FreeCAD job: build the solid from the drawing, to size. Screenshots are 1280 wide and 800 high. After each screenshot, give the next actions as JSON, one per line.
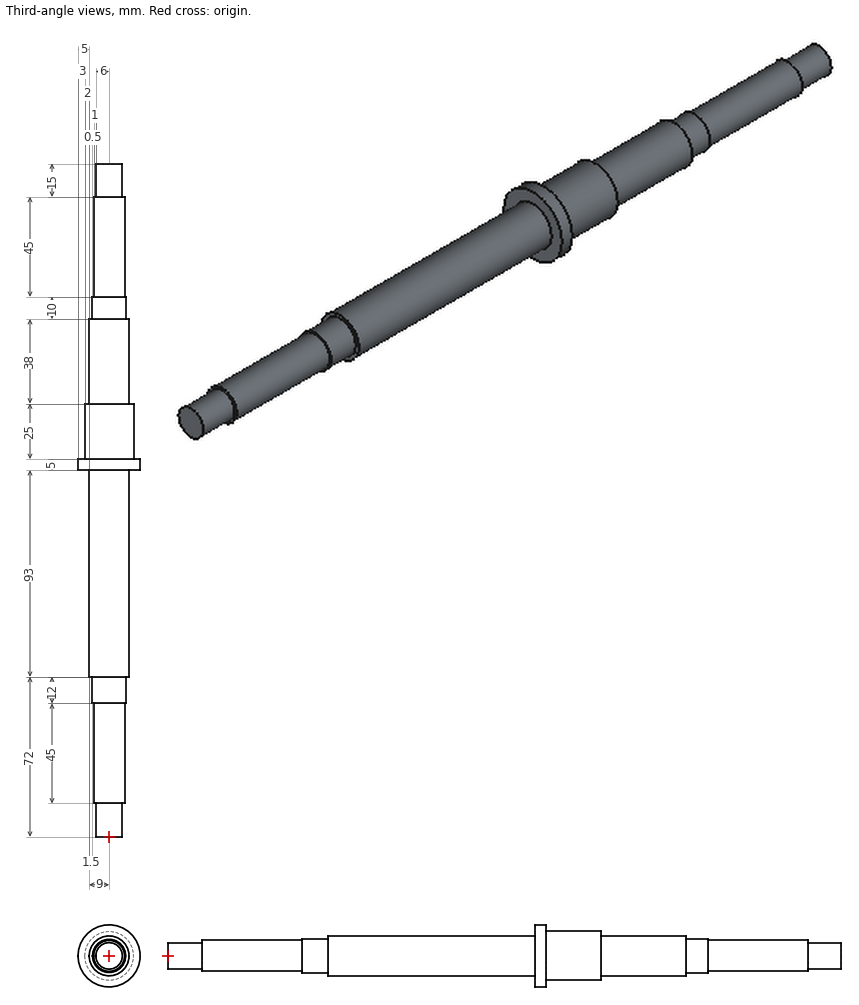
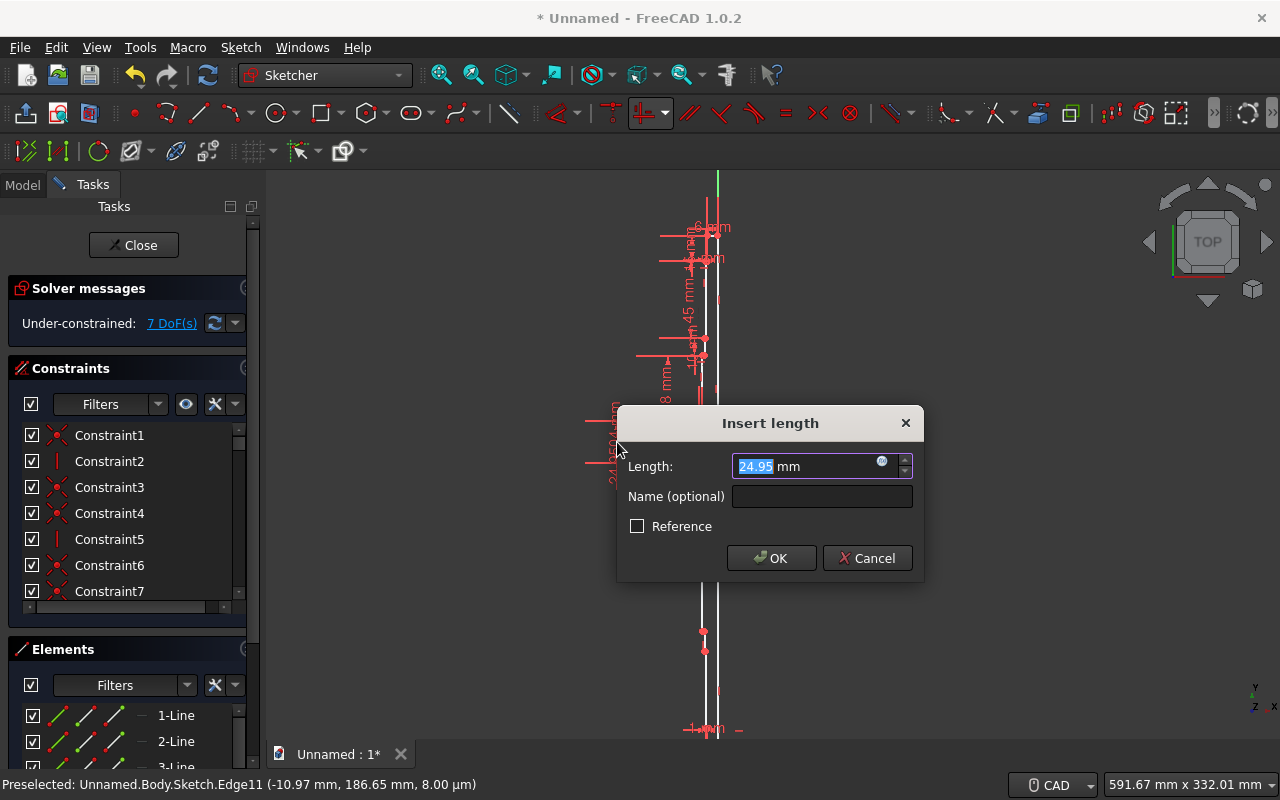
{"action": "type", "text": "25"}
{"action": "key", "text": "Return"}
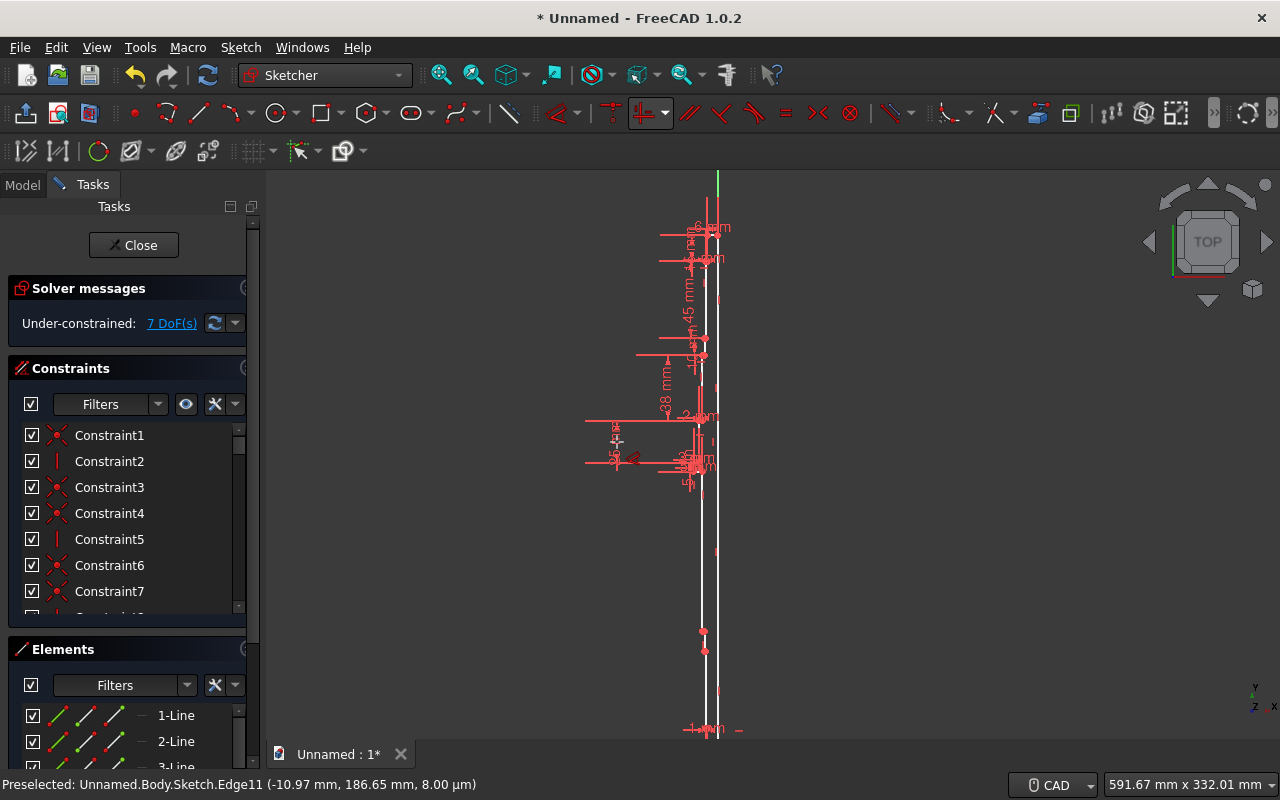
{"action": "left_click", "coordinate": [702, 520]}
{"action": "left_click", "coordinate": [668, 552]}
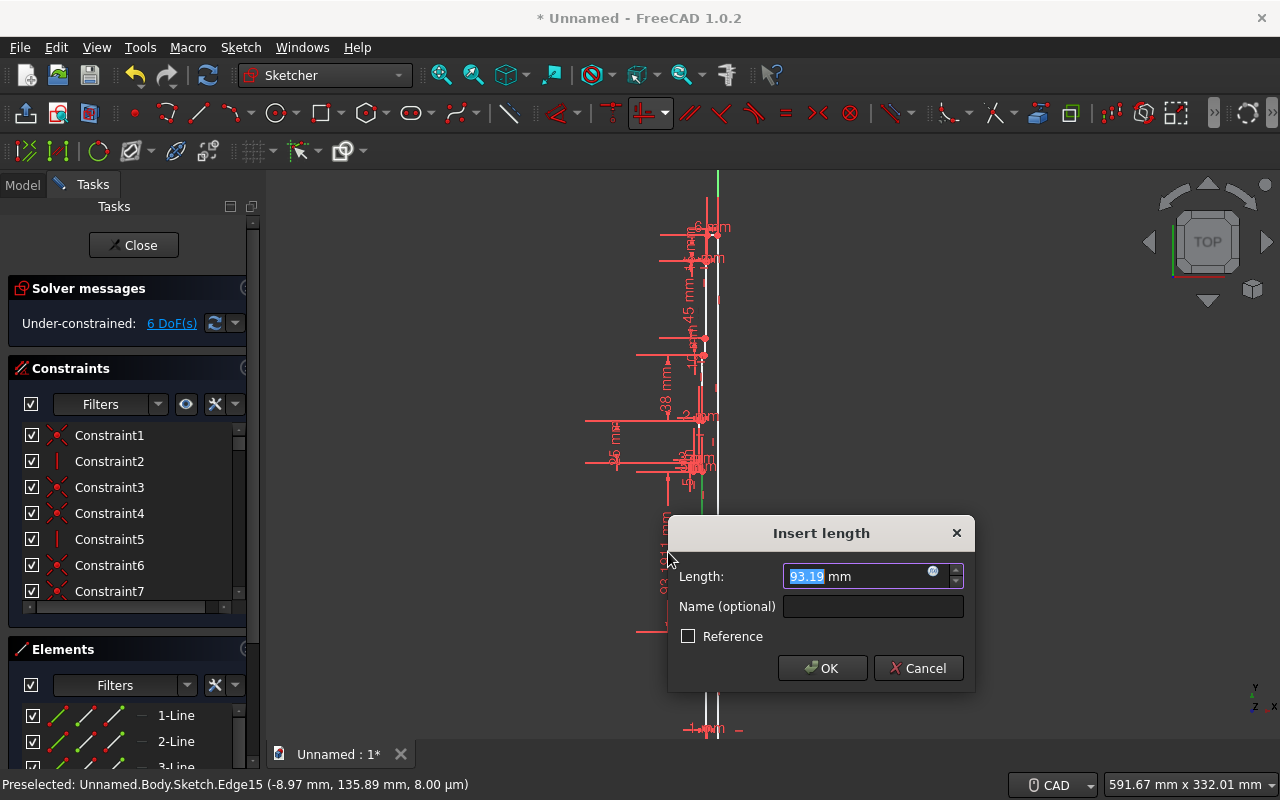
{"action": "type", "text": "93"}
{"action": "key", "text": "Return"}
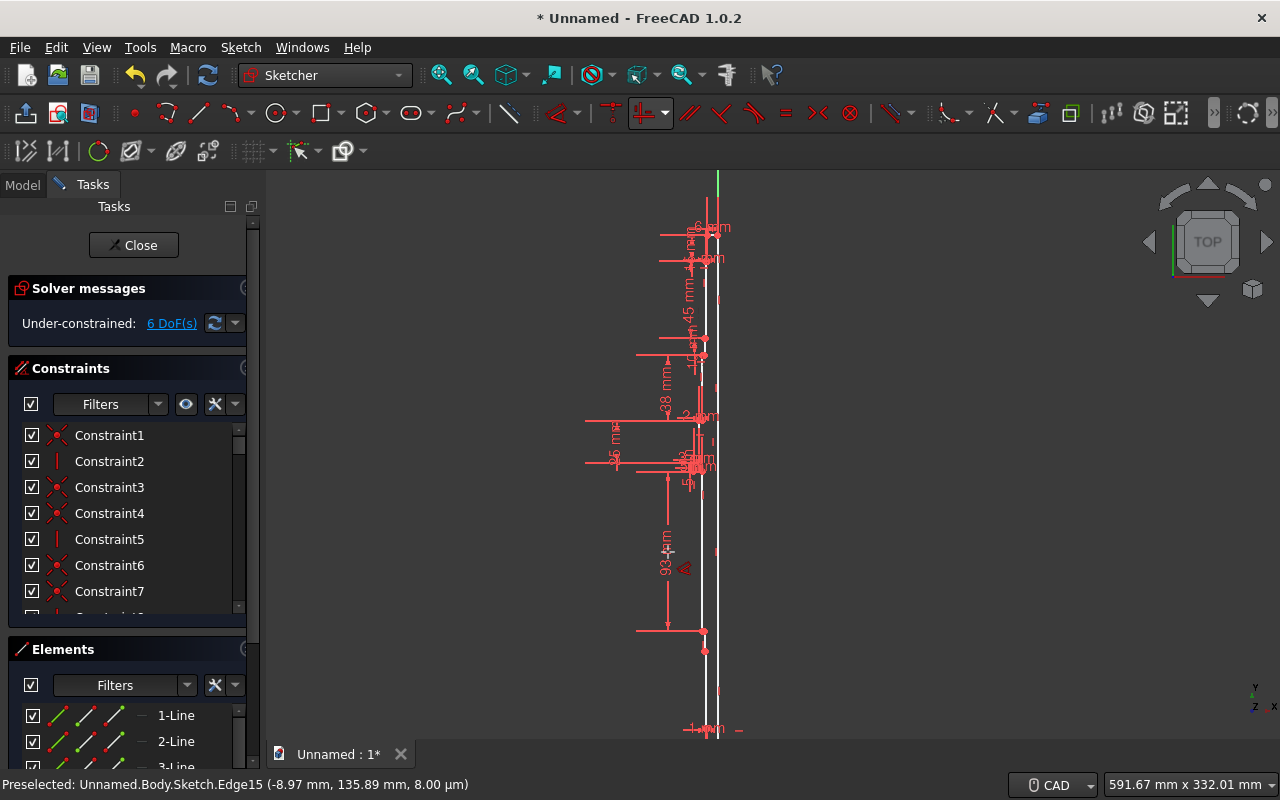
{"action": "scroll", "coordinate": [705, 642], "scroll_direction": "up", "scroll_amount": 4}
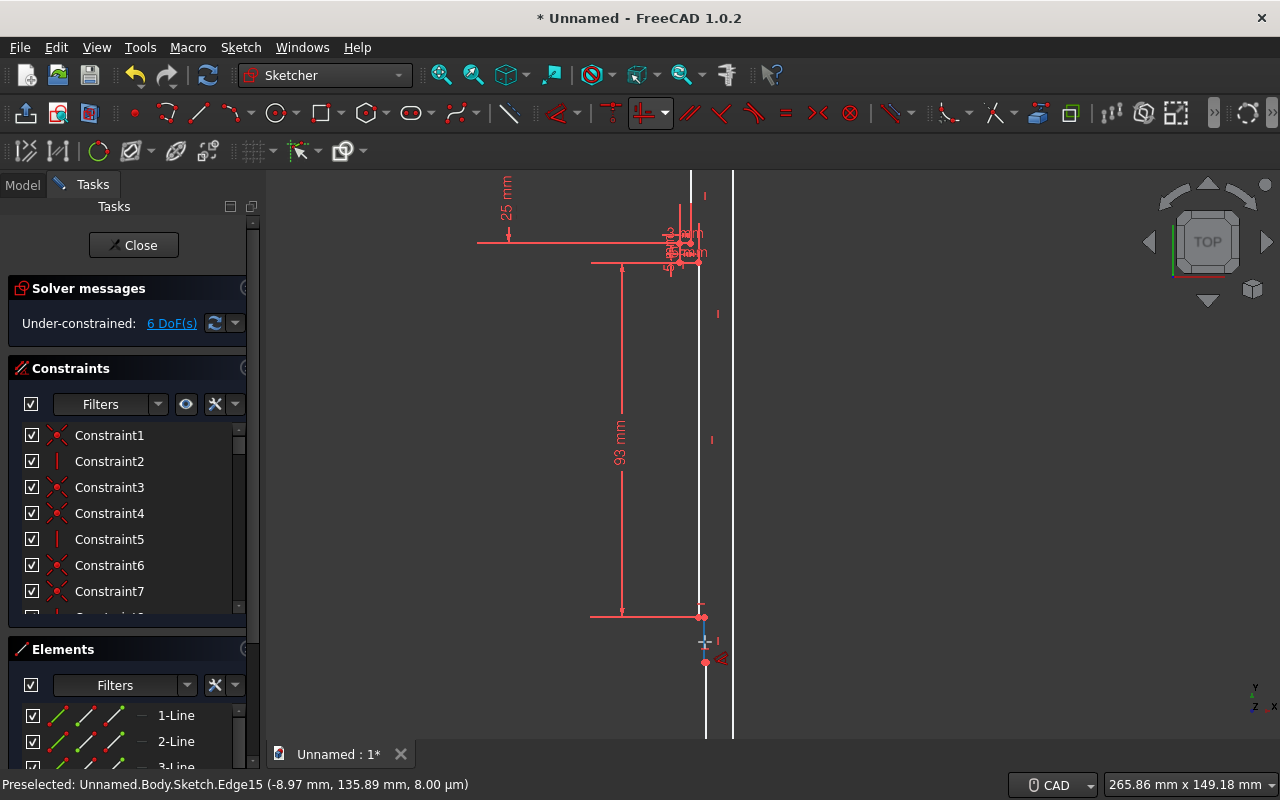
{"action": "left_click", "coordinate": [704, 640]}
{"action": "left_click", "coordinate": [670, 640]}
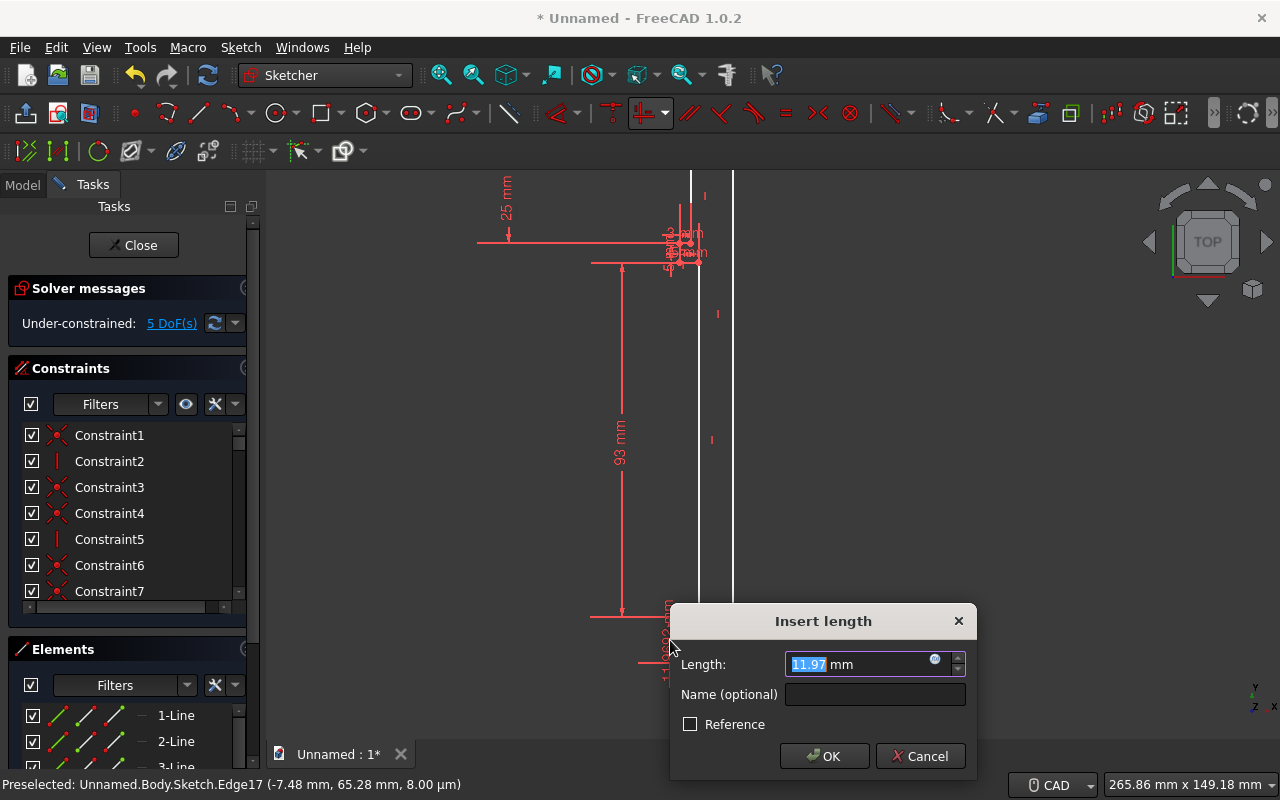
{"action": "type", "text": "12"}
{"action": "key", "text": "Return"}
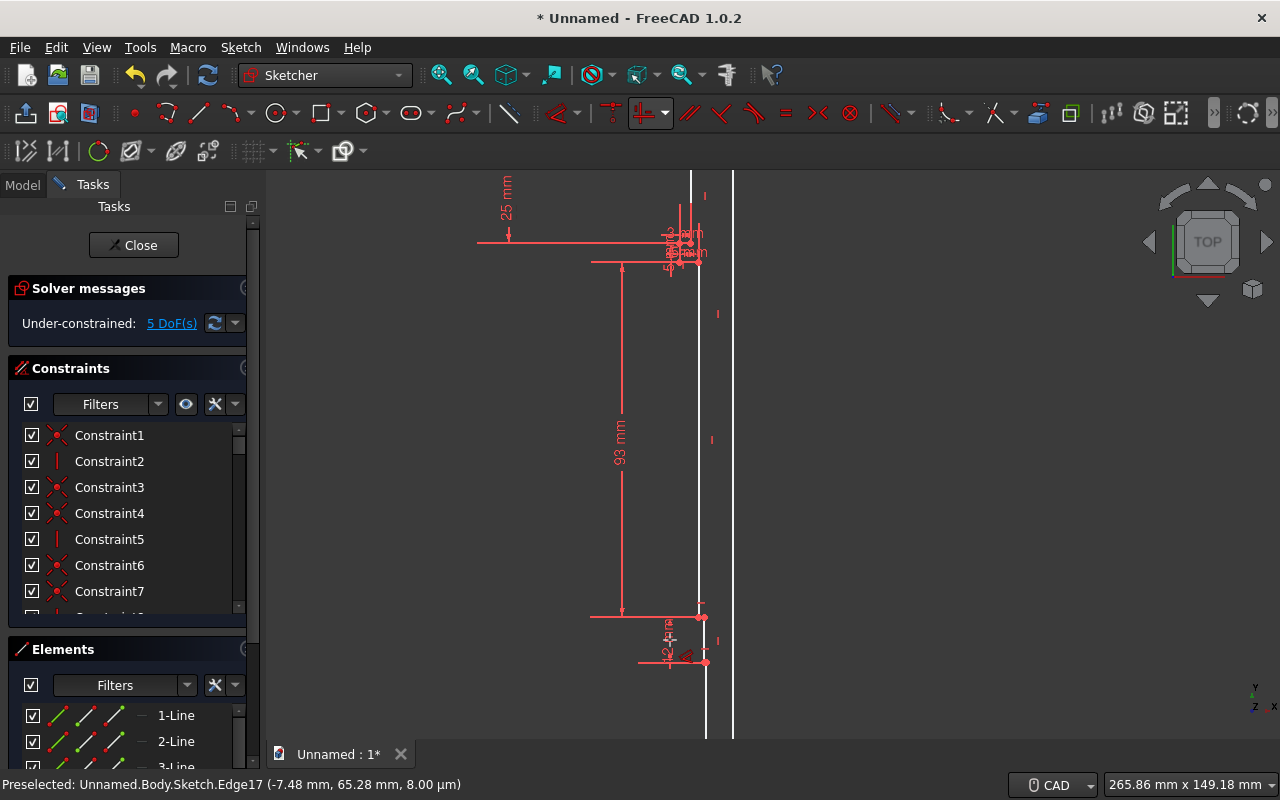
{"action": "left_click", "coordinate": [706, 697]}
{"action": "left_click", "coordinate": [672, 687]}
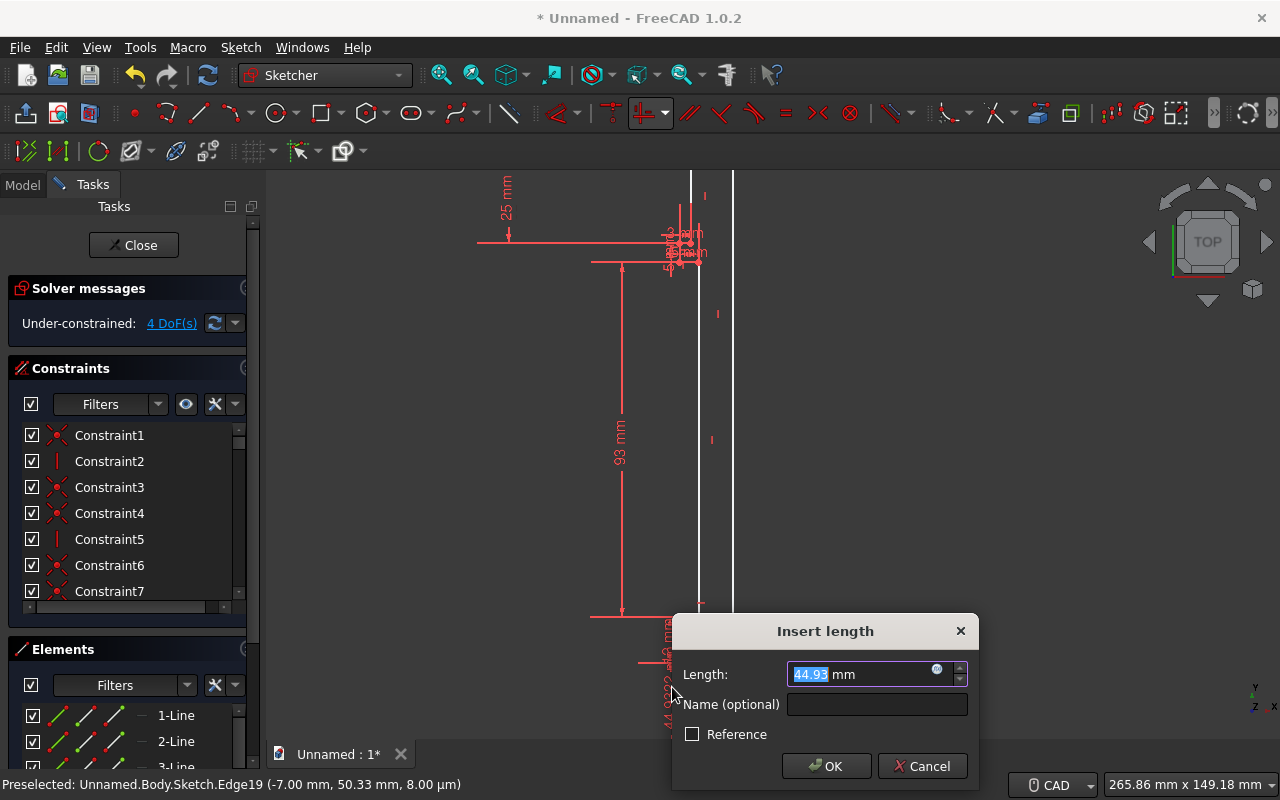
{"action": "type", "text": "45"}
{"action": "key", "text": "Return"}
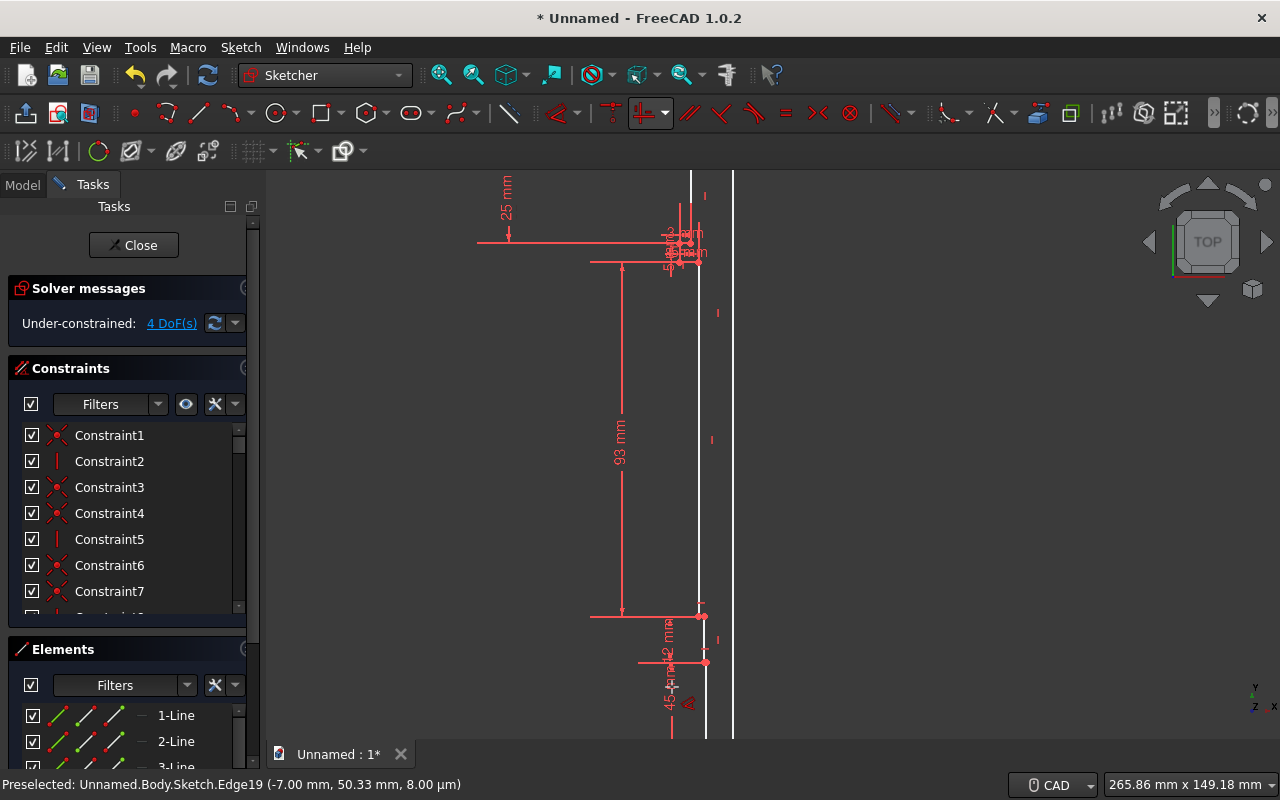
{"action": "scroll", "coordinate": [704, 516], "scroll_direction": "down", "scroll_amount": 6}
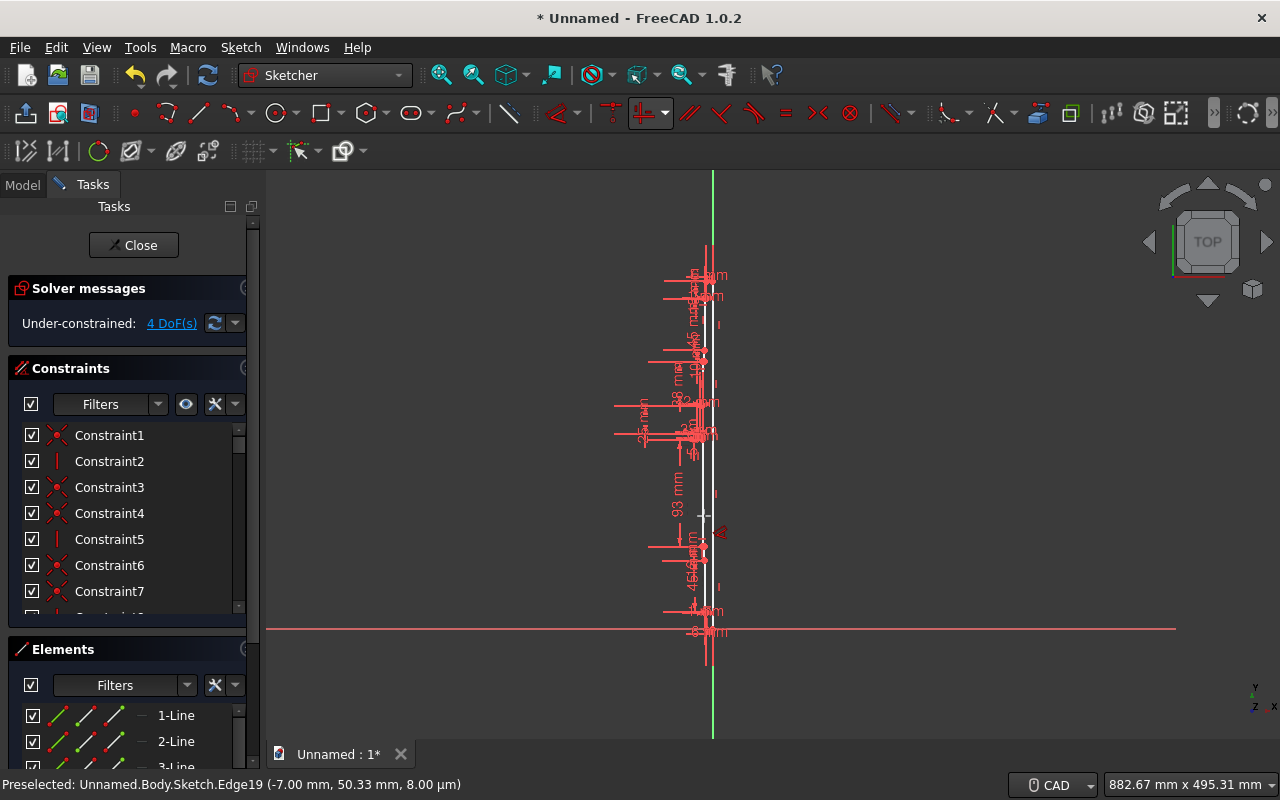
{"action": "scroll", "coordinate": [703, 362], "scroll_direction": "up", "scroll_amount": 10}